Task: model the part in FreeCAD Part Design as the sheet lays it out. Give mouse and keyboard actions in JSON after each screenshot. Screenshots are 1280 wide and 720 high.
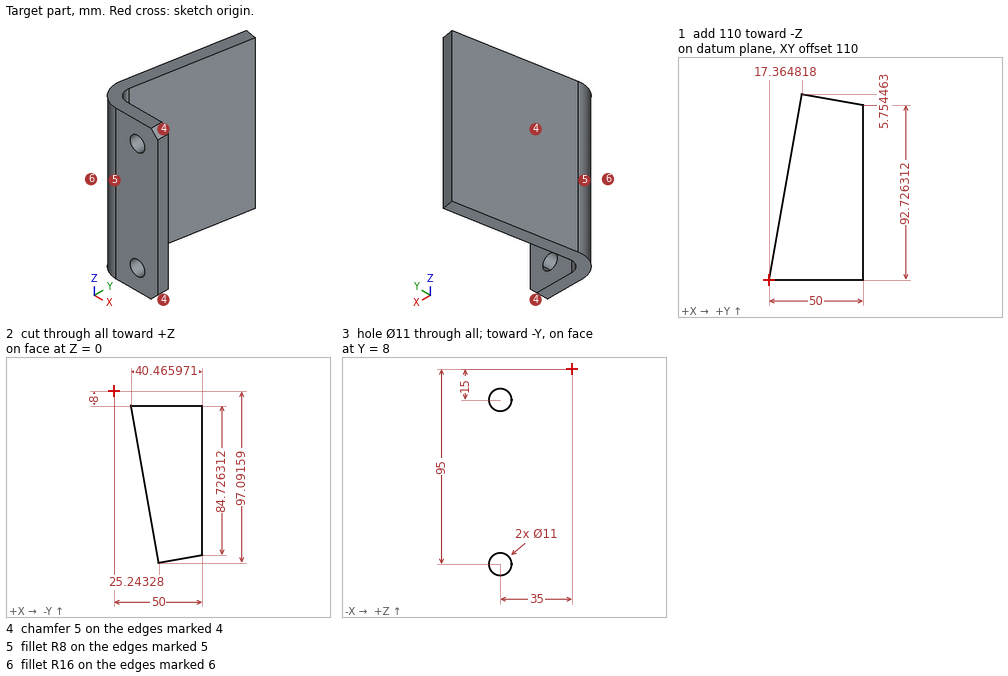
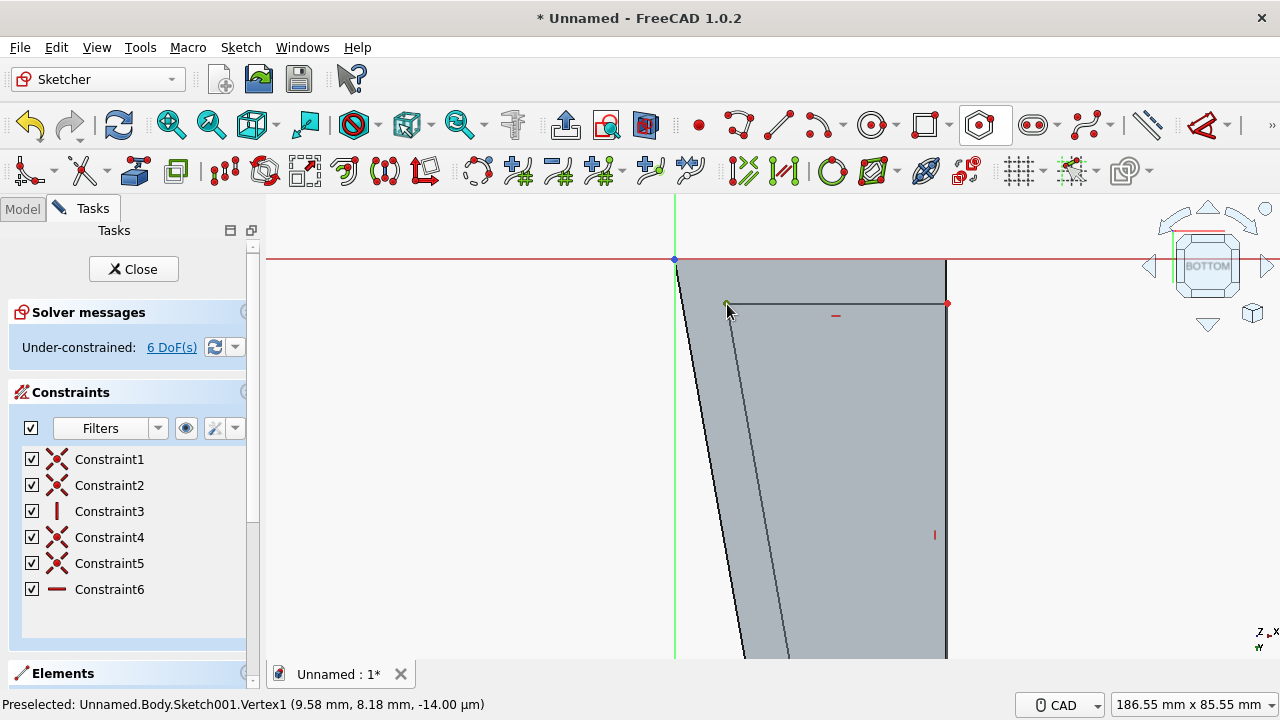
{"action": "key", "text": "i"}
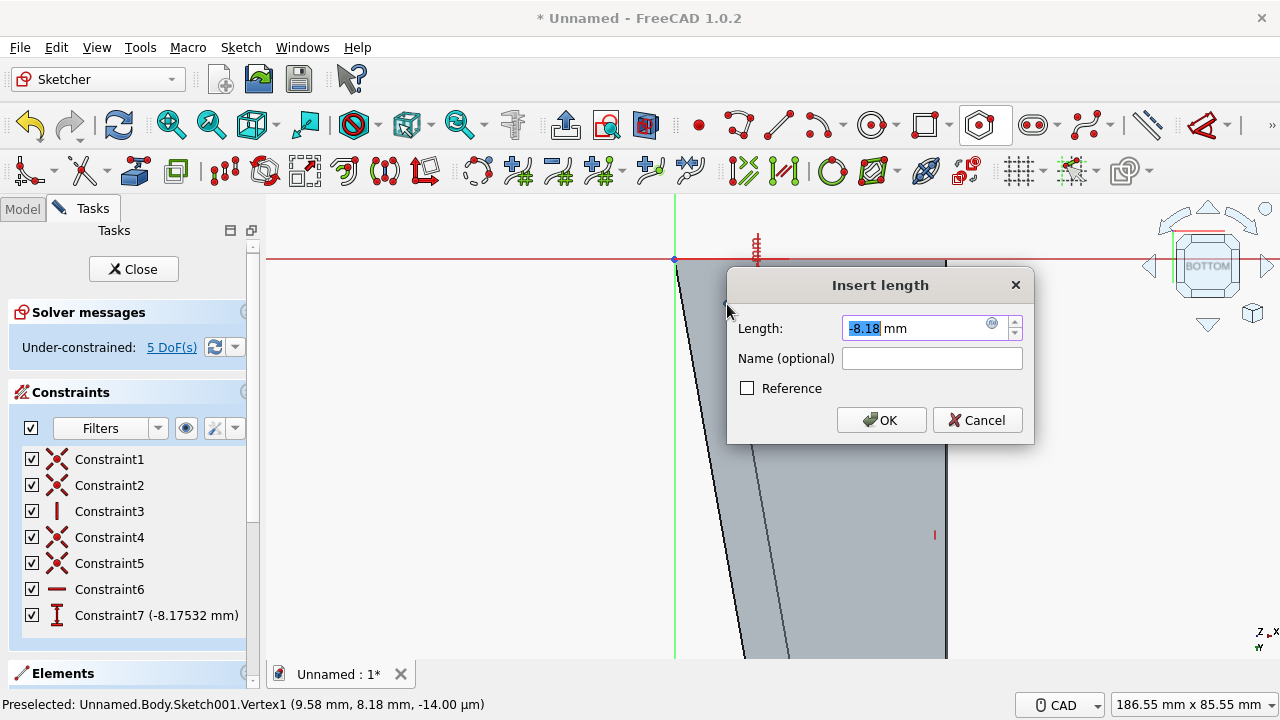
{"action": "type", "text": "-8"}
{"action": "key", "text": "Return"}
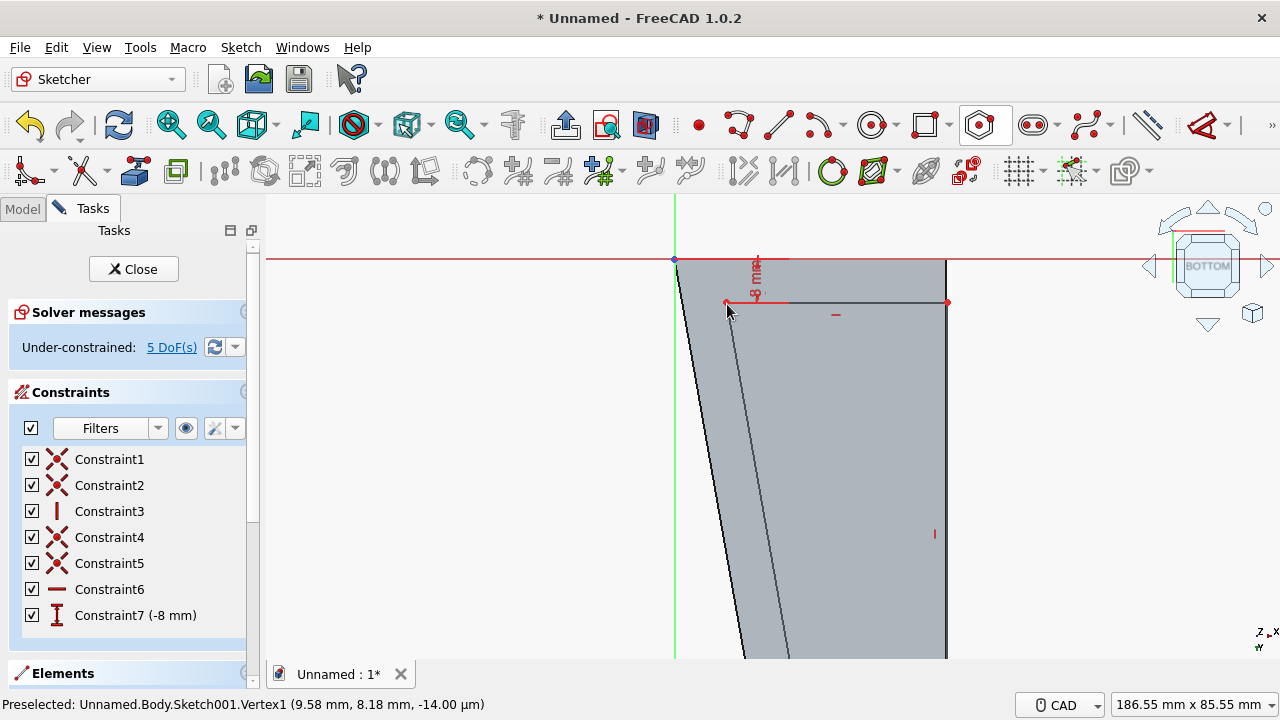
{"action": "scroll", "coordinate": [576, 309], "scroll_direction": "down", "scroll_amount": 3}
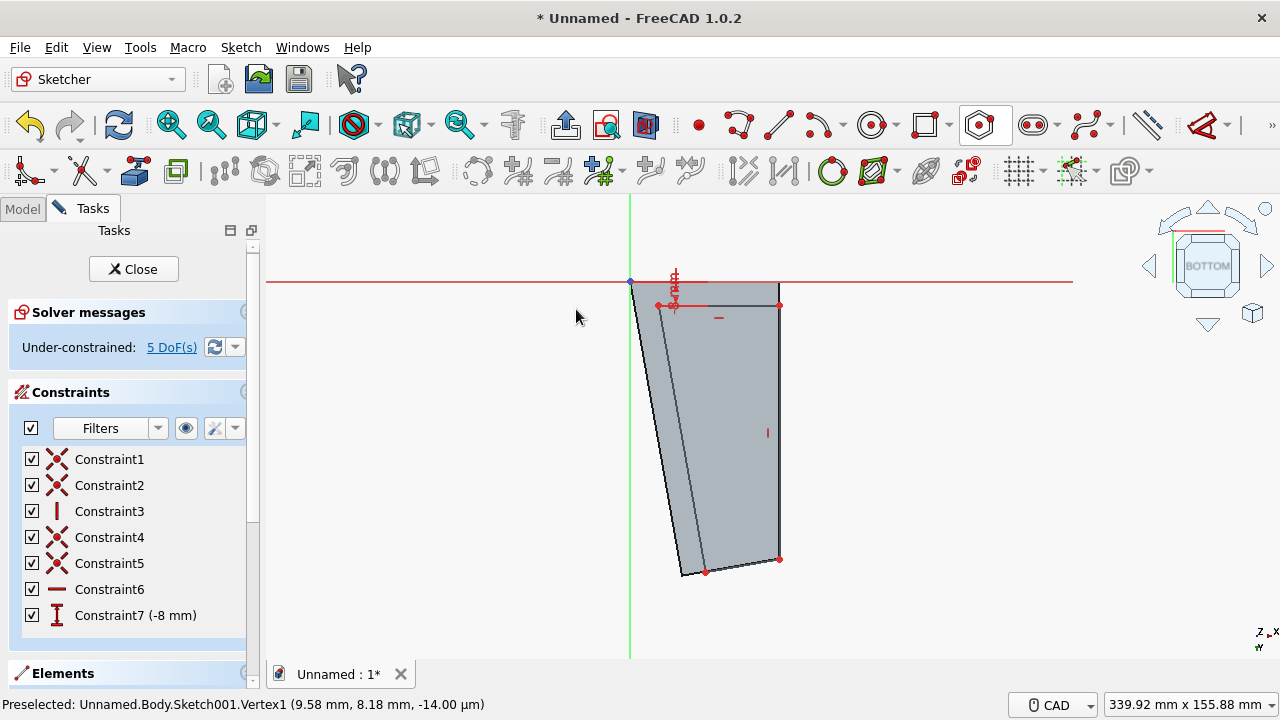
{"action": "left_click", "coordinate": [780, 559]}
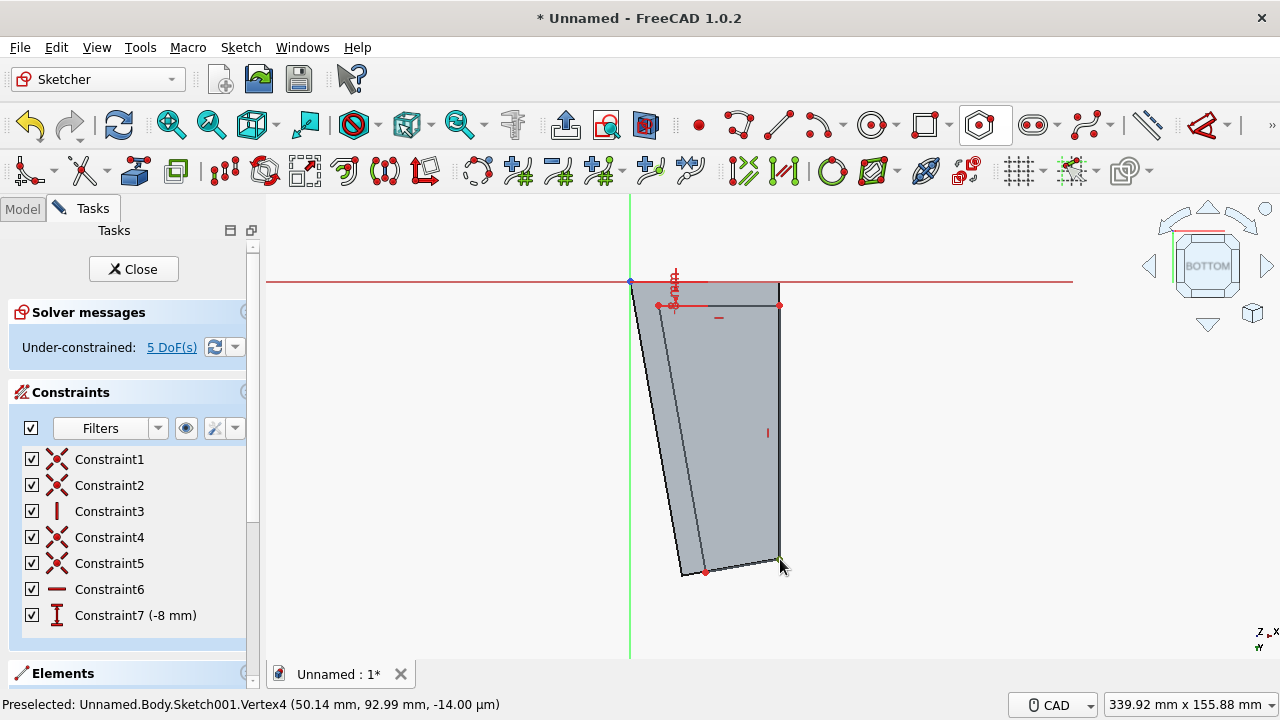
{"action": "key", "text": "l"}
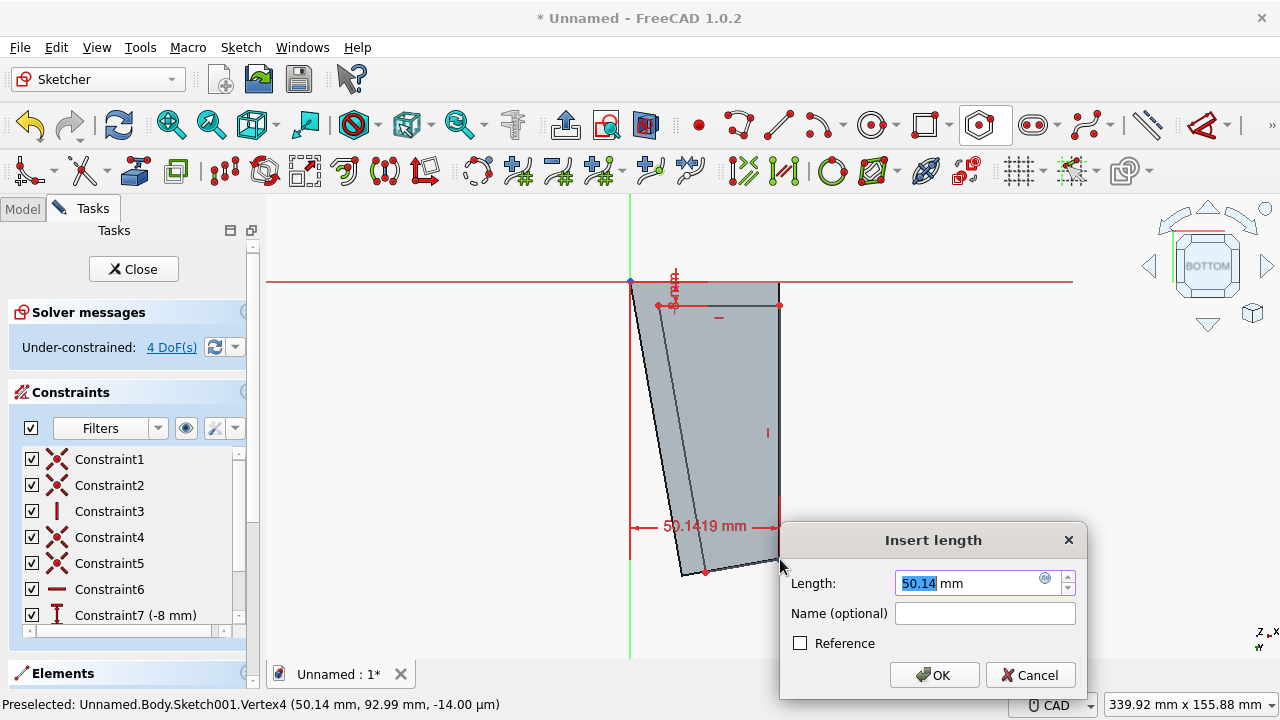
{"action": "type", "text": "50"}
{"action": "key", "text": "Return"}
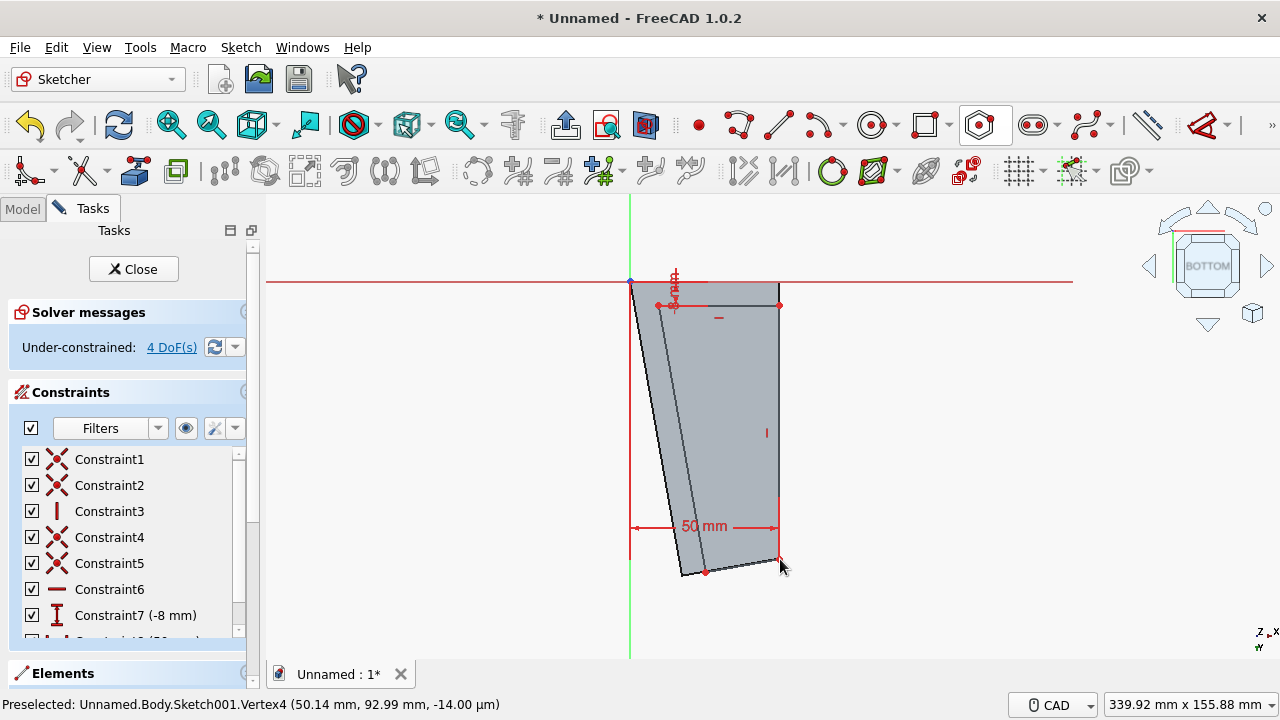
{"action": "left_click", "coordinate": [779, 483]}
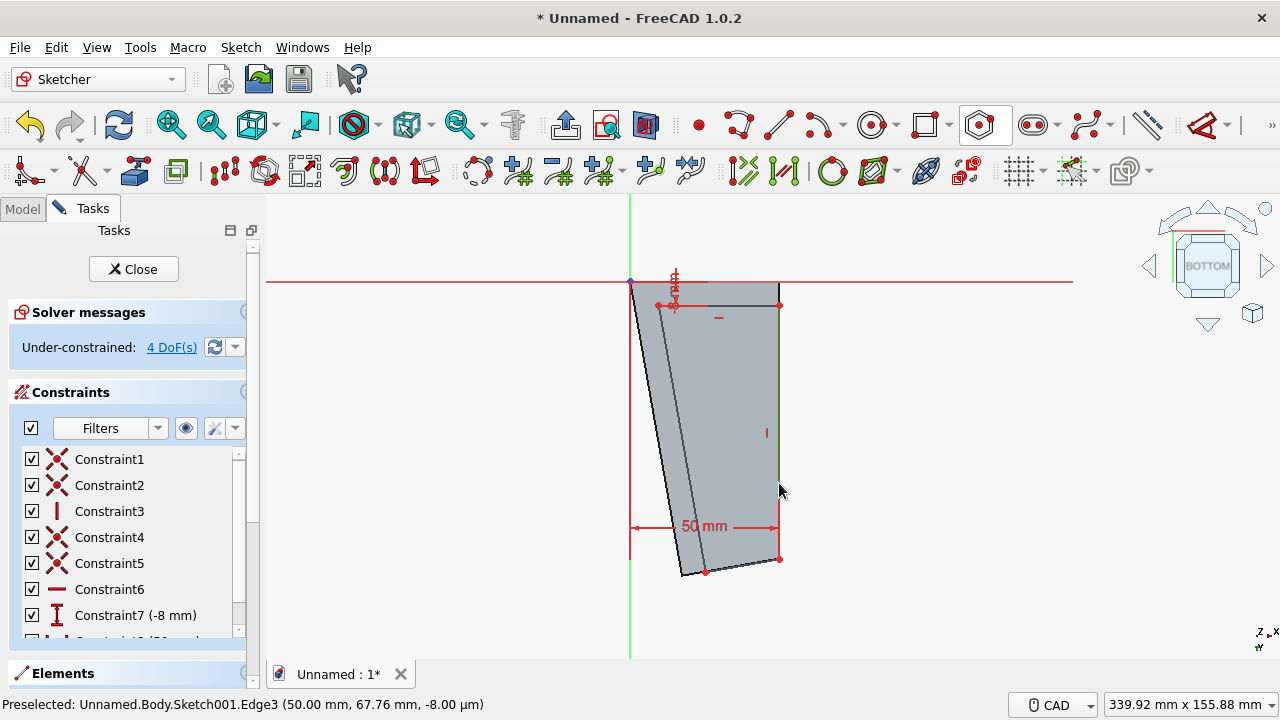
{"action": "left_click", "coordinate": [1230, 126]}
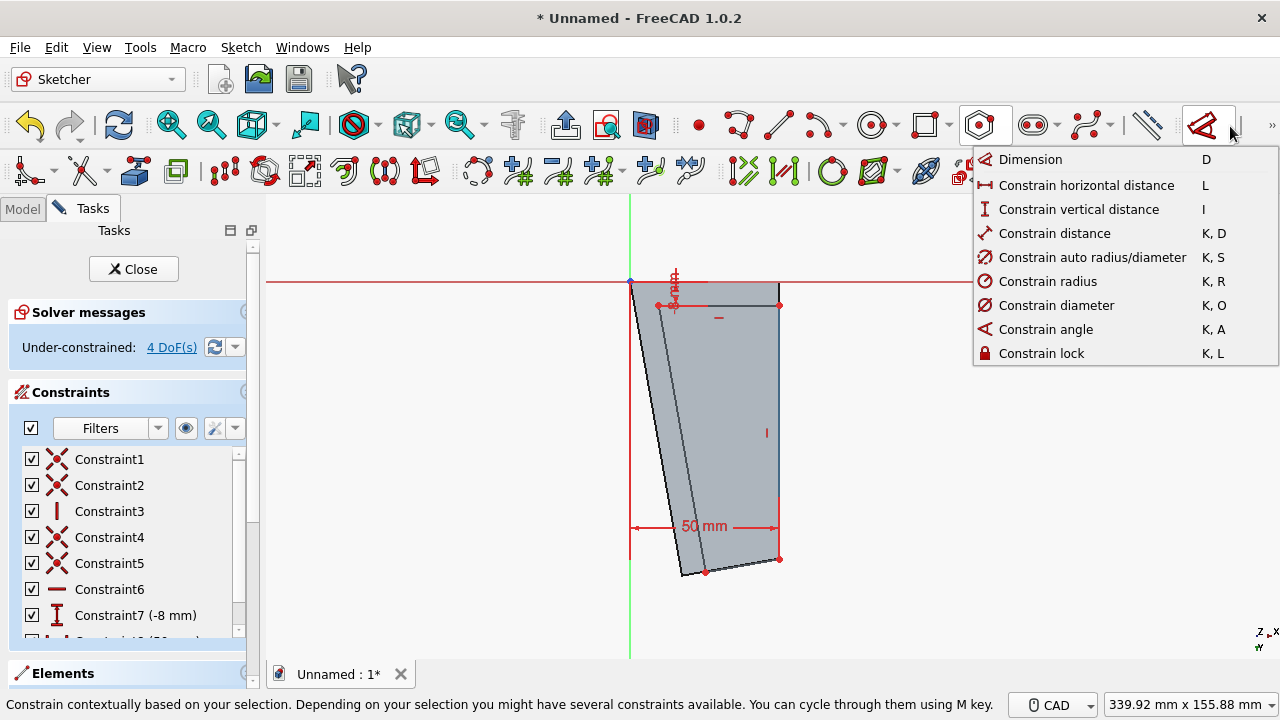
{"action": "left_click", "coordinate": [1126, 209]}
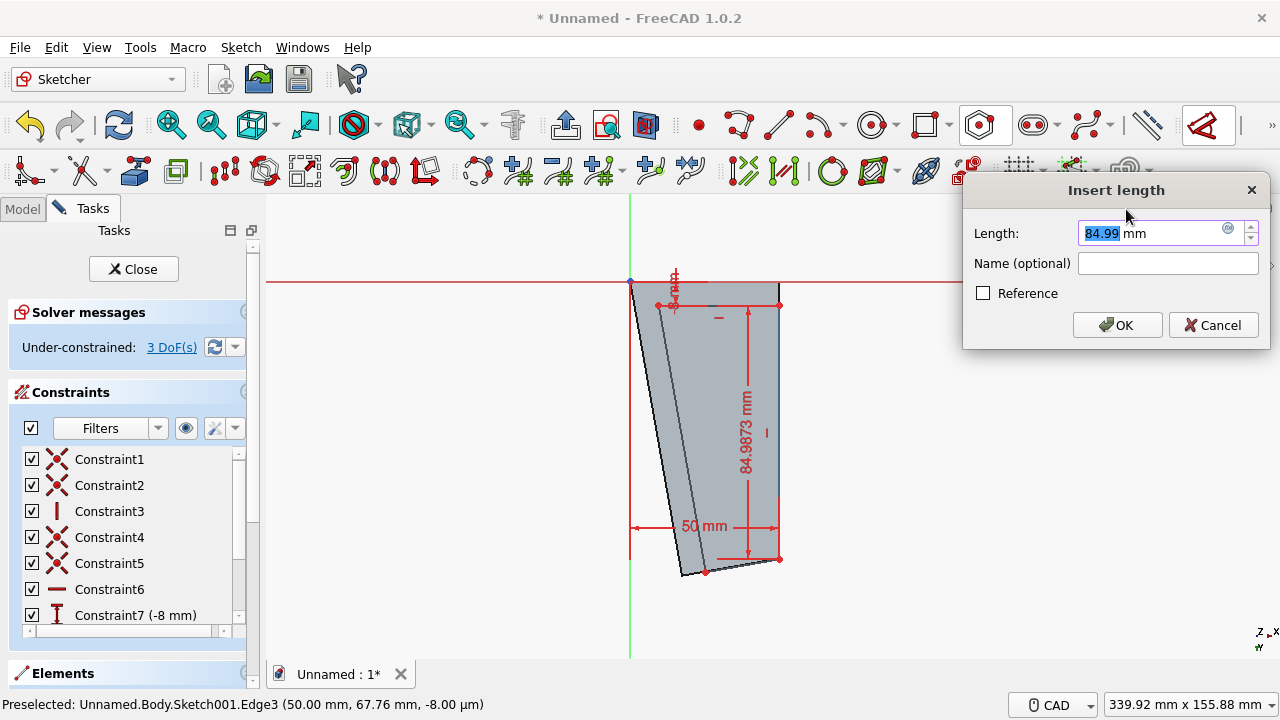
{"action": "type", "text": "84.726312"}
{"action": "key", "text": "Return"}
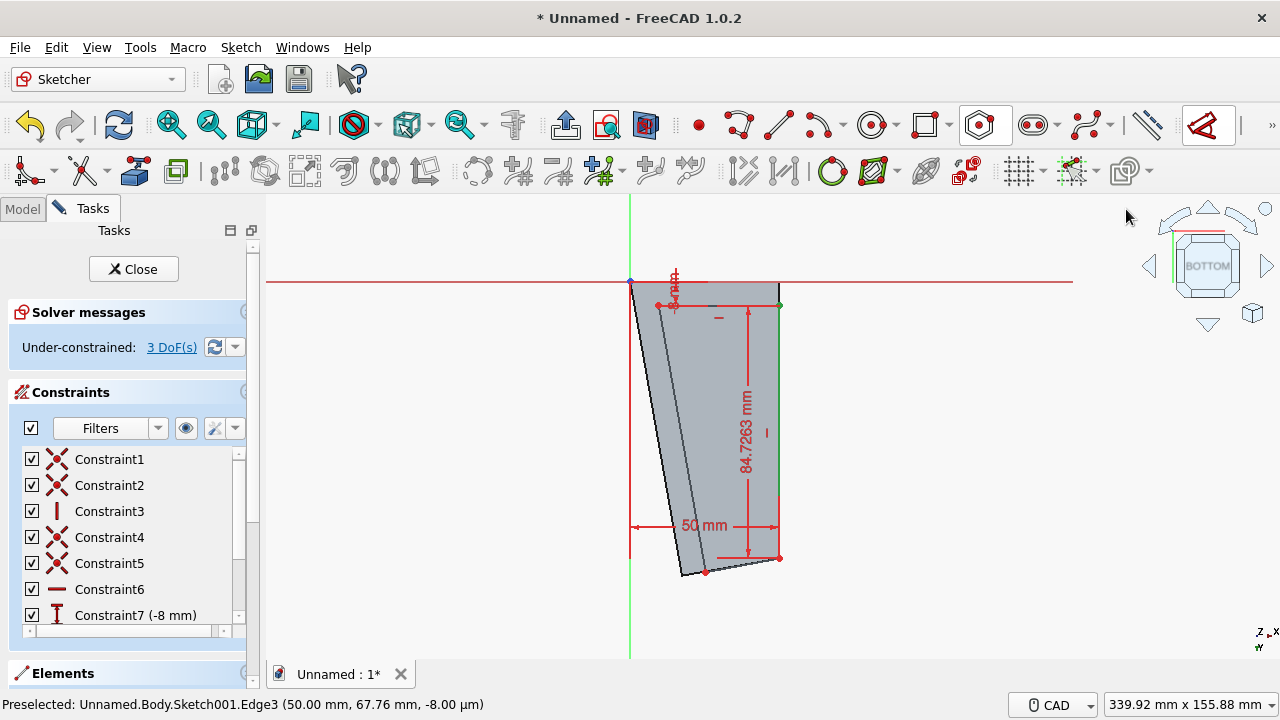
{"action": "left_click", "coordinate": [743, 306]}